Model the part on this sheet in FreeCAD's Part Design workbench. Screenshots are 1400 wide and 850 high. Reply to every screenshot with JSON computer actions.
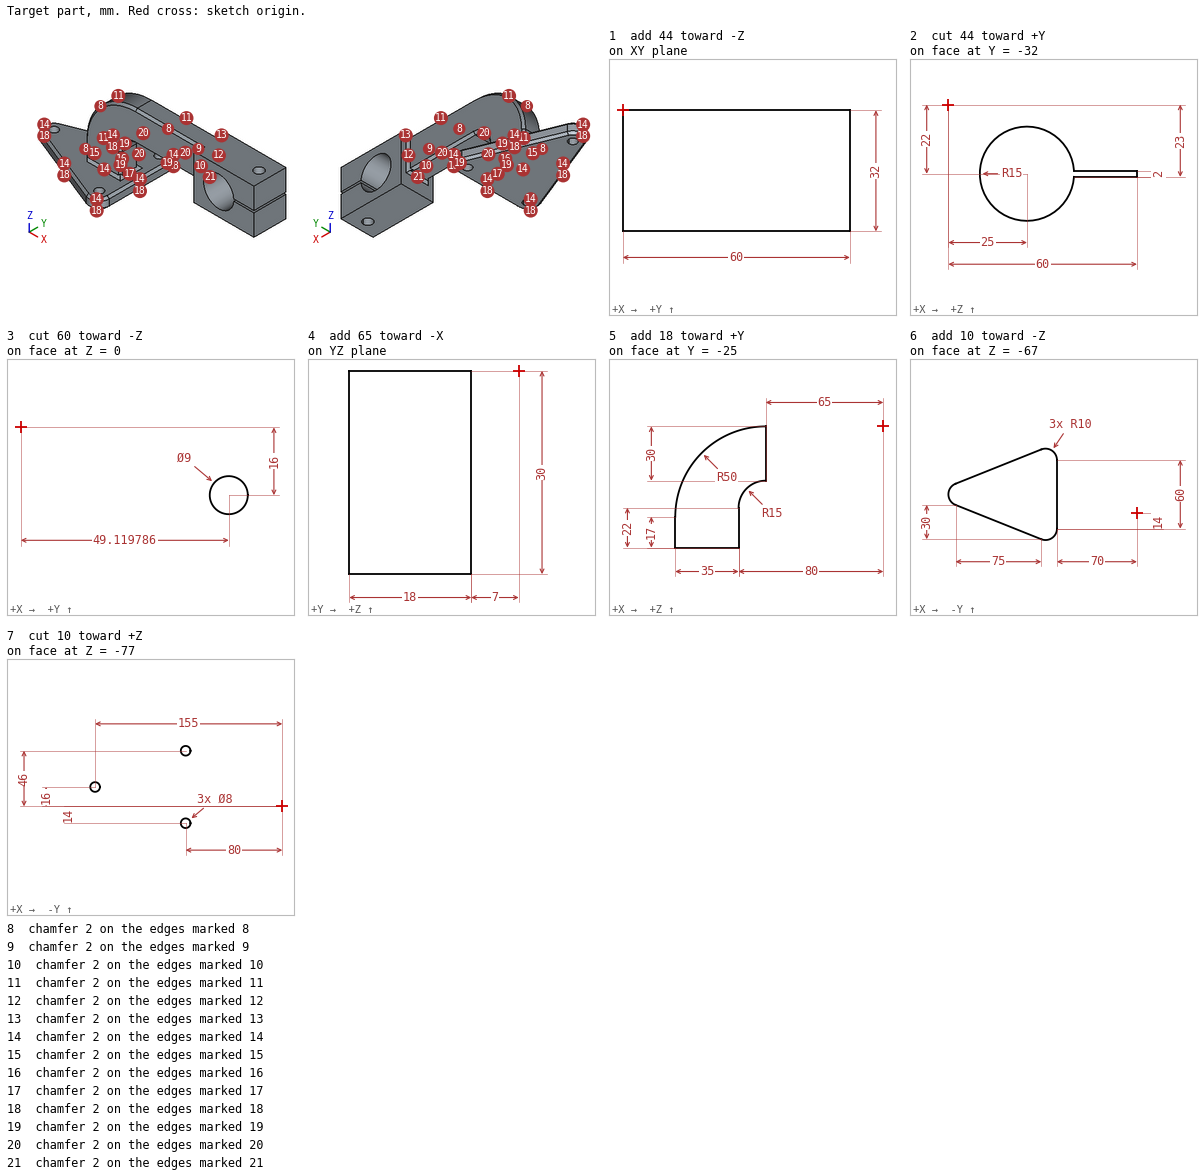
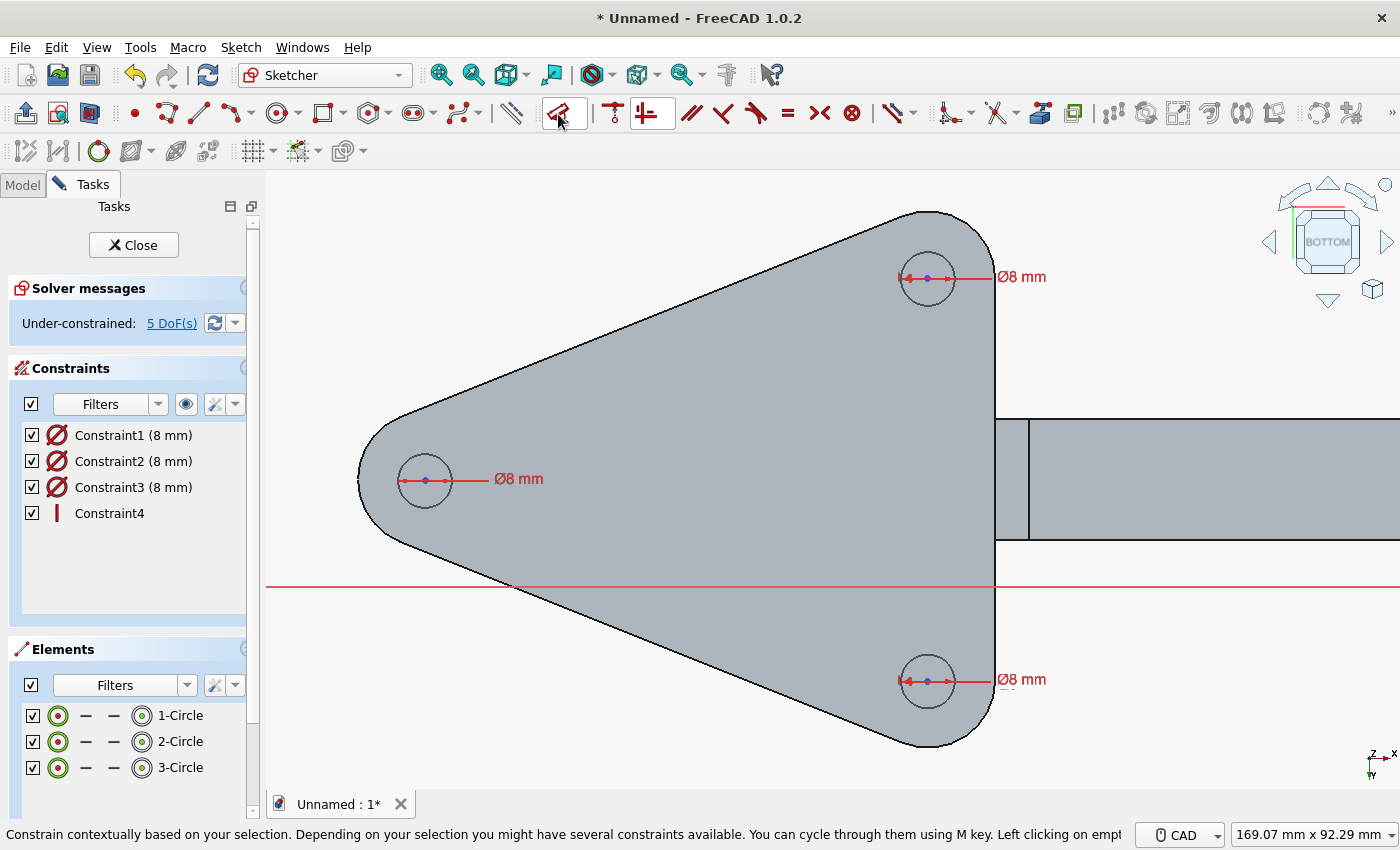
{"action": "left_click", "coordinate": [928, 682]}
{"action": "left_click", "coordinate": [1081, 716]}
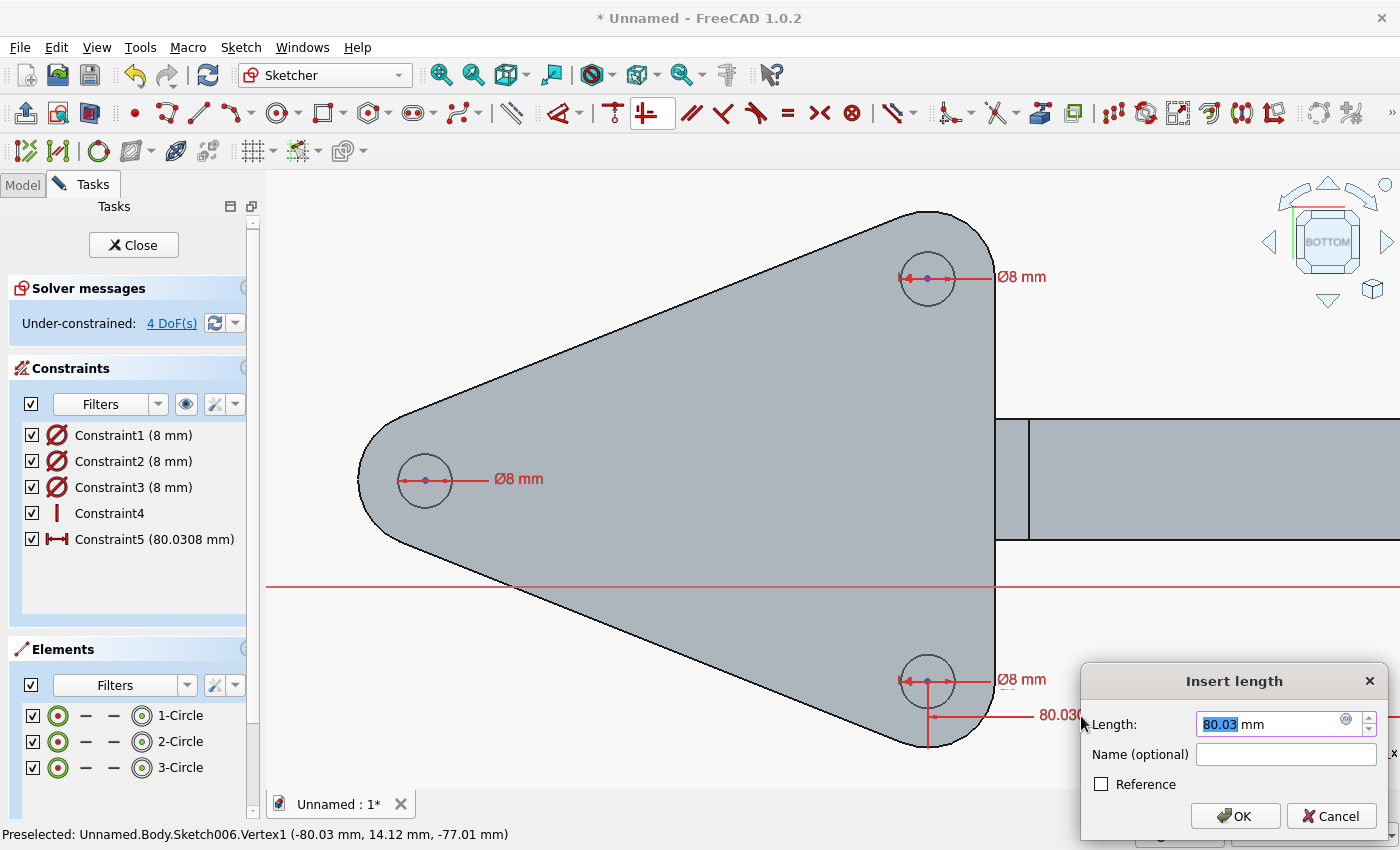
{"action": "type", "text": "80"}
{"action": "key", "text": "Return"}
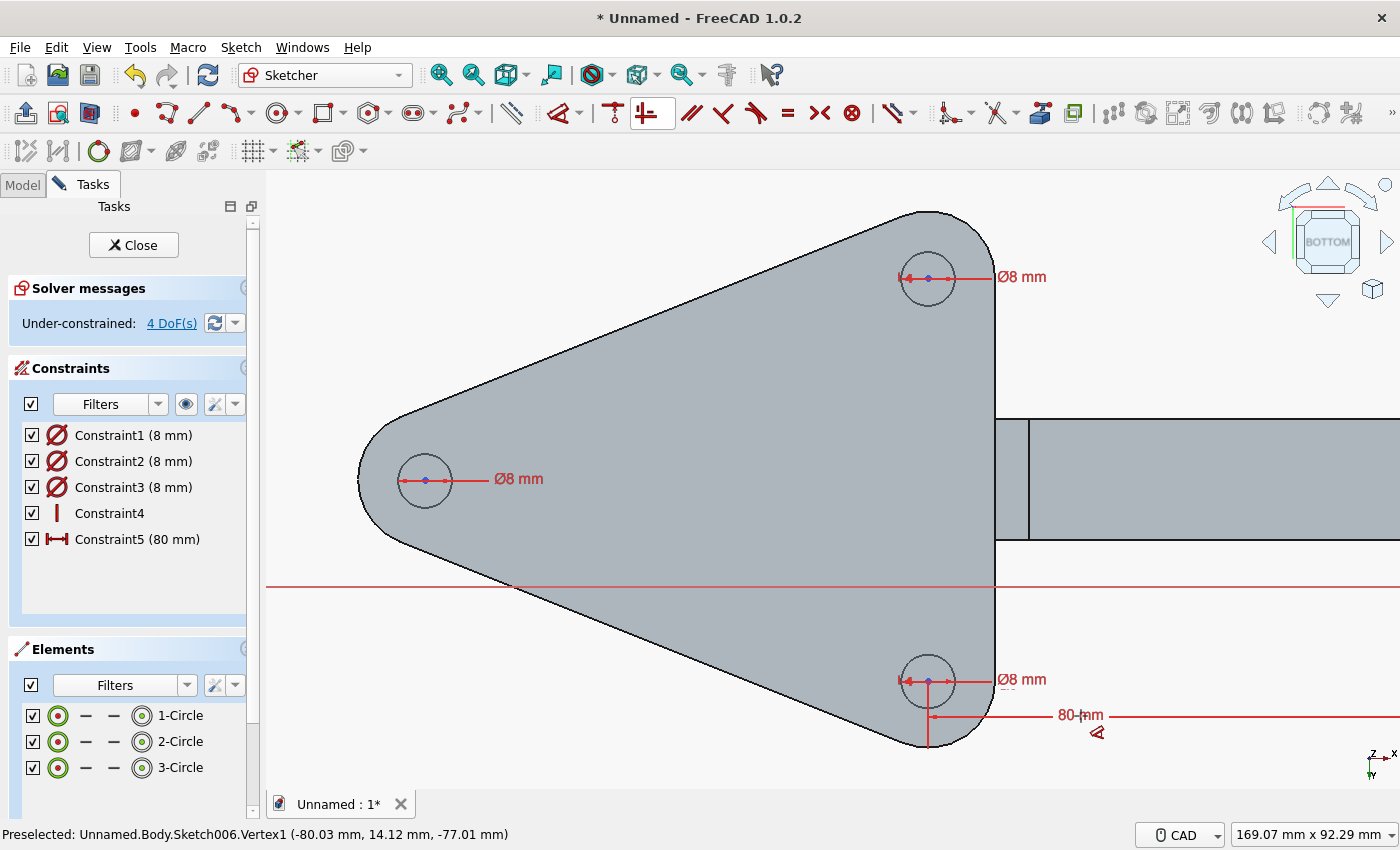
{"action": "left_click", "coordinate": [928, 682]}
{"action": "left_click", "coordinate": [894, 634]}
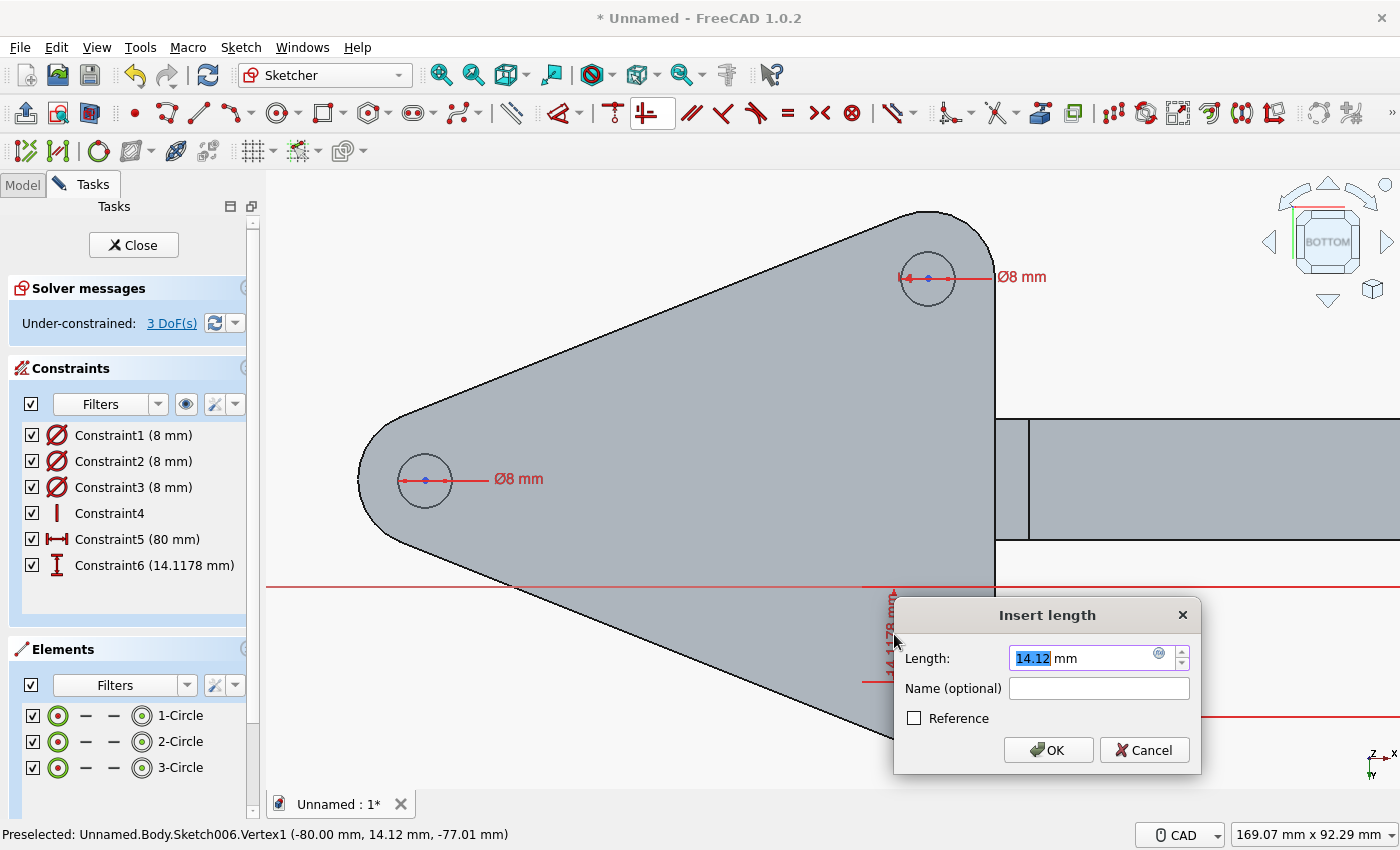
{"action": "type", "text": "14"}
{"action": "key", "text": "Return"}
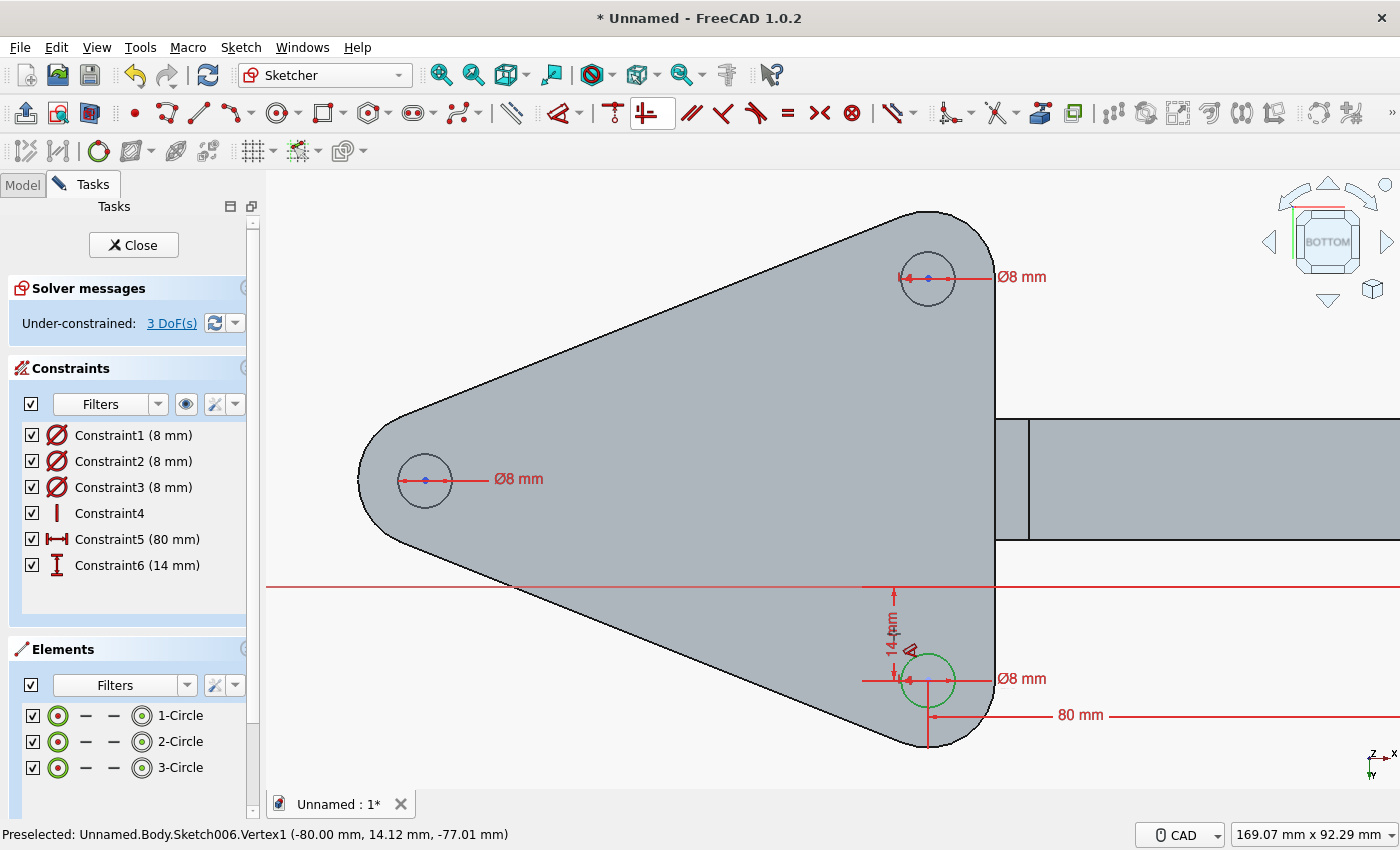
{"action": "left_click", "coordinate": [425, 481]}
{"action": "left_click", "coordinate": [391, 534]}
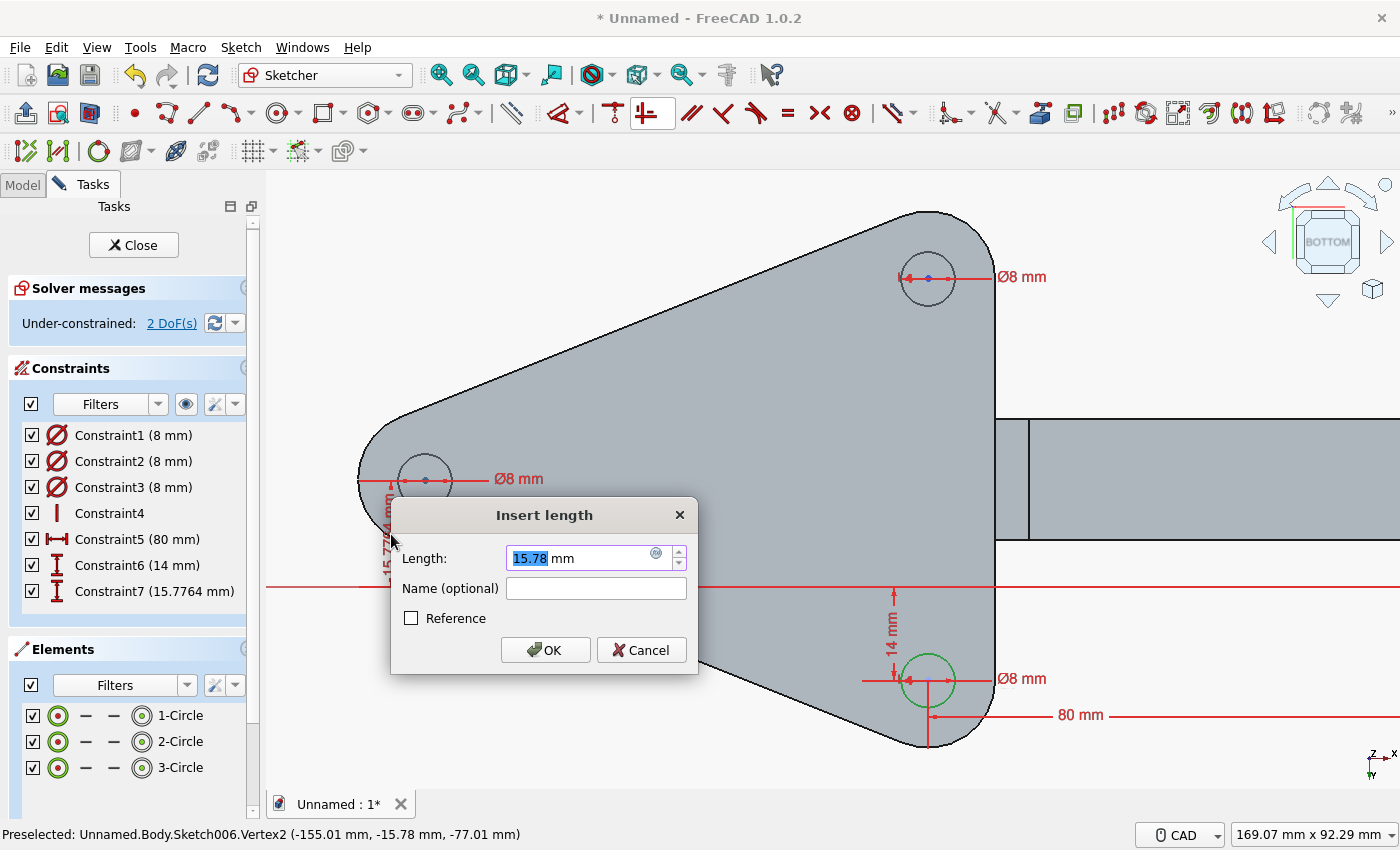
{"action": "type", "text": "16"}
{"action": "key", "text": "Return"}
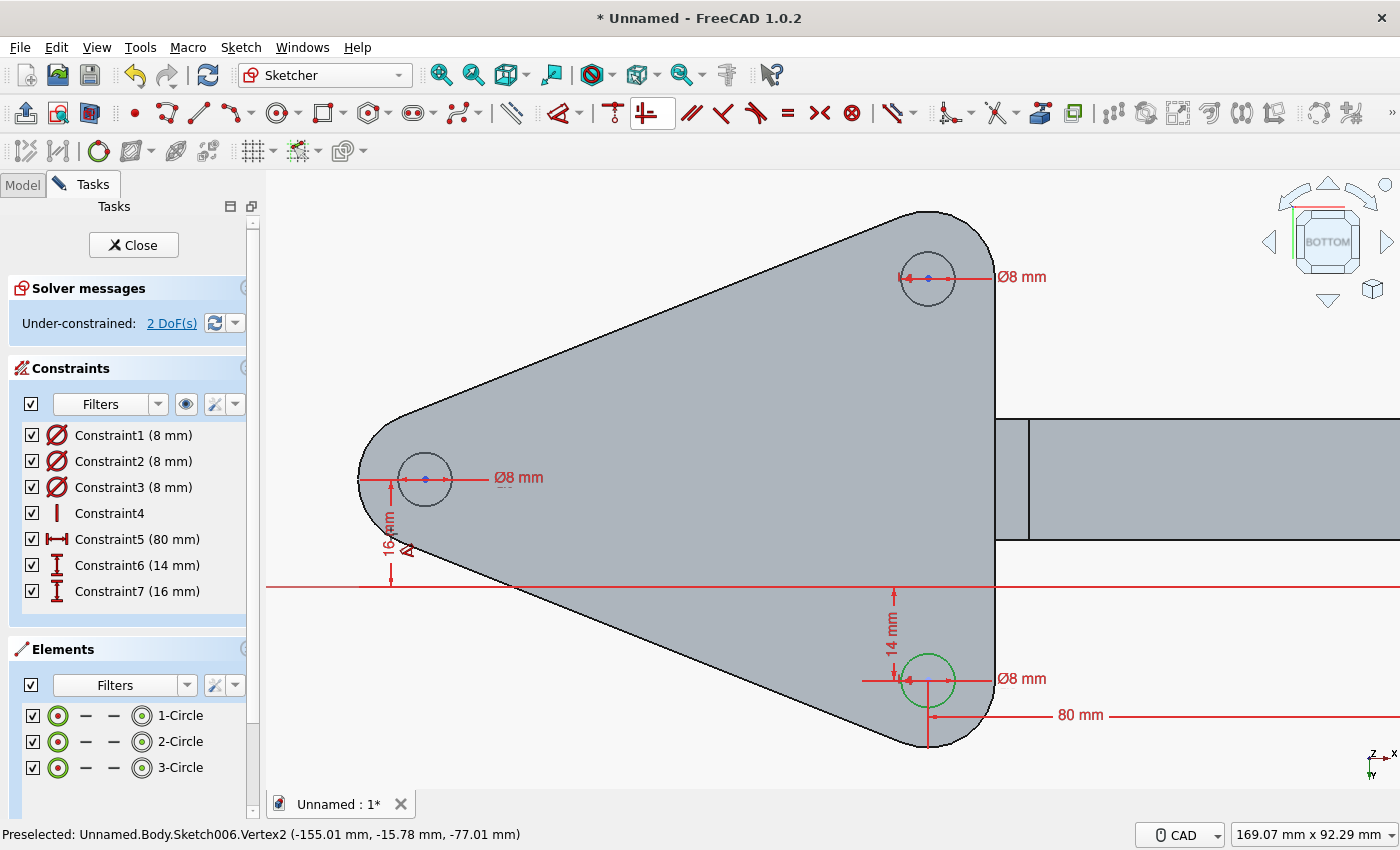
{"action": "left_click", "coordinate": [928, 279]}
{"action": "left_click", "coordinate": [894, 433]}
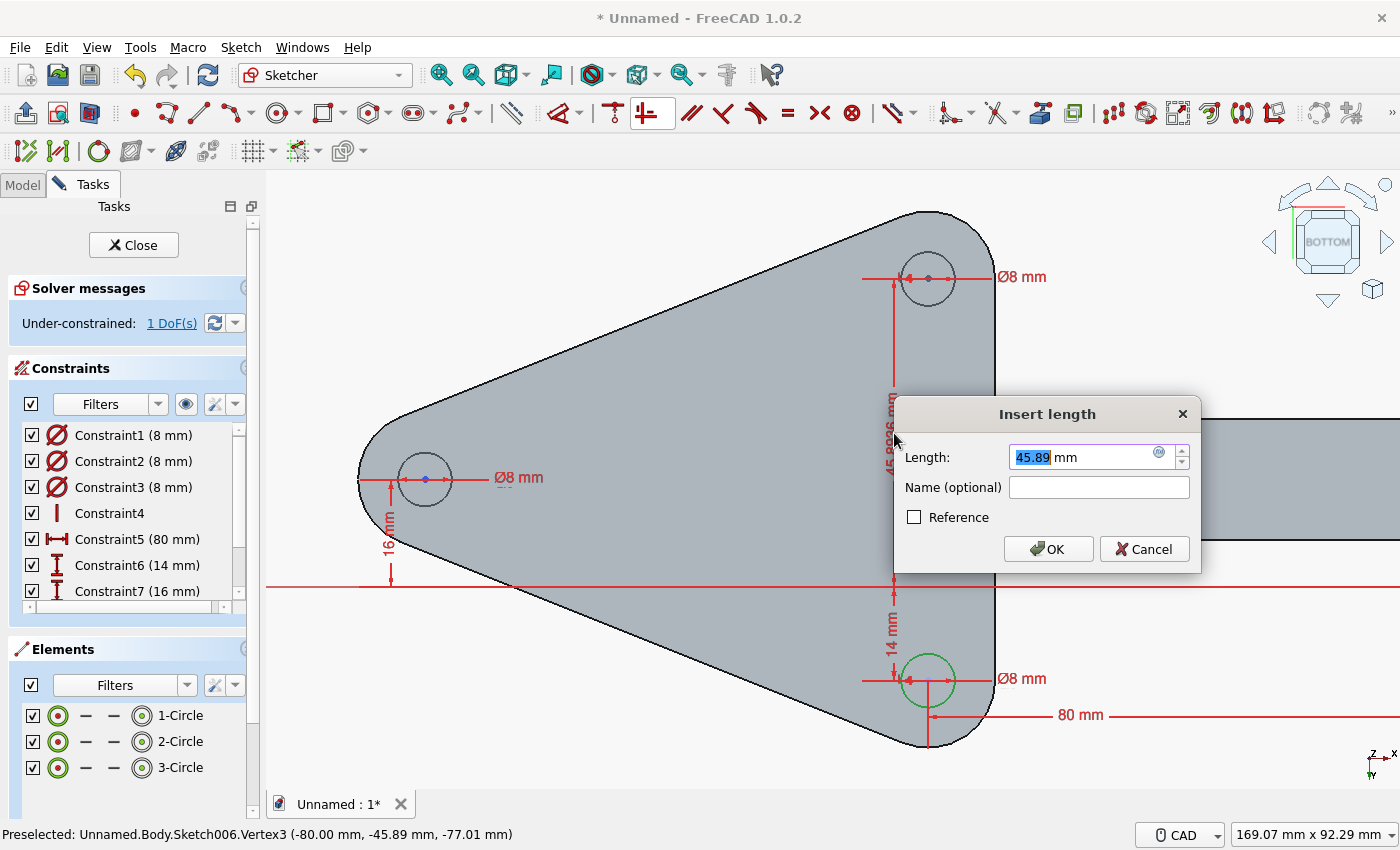
{"action": "type", "text": "46"}
{"action": "key", "text": "Return"}